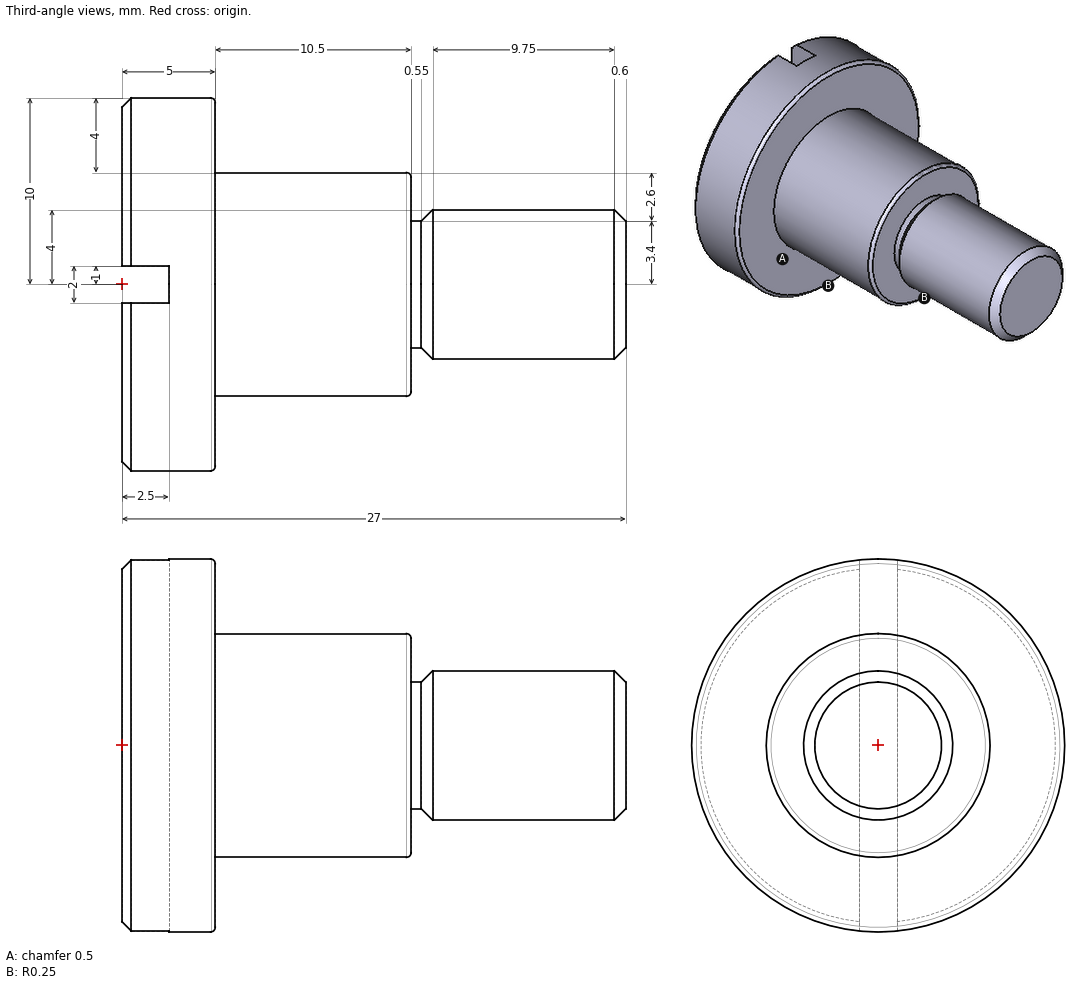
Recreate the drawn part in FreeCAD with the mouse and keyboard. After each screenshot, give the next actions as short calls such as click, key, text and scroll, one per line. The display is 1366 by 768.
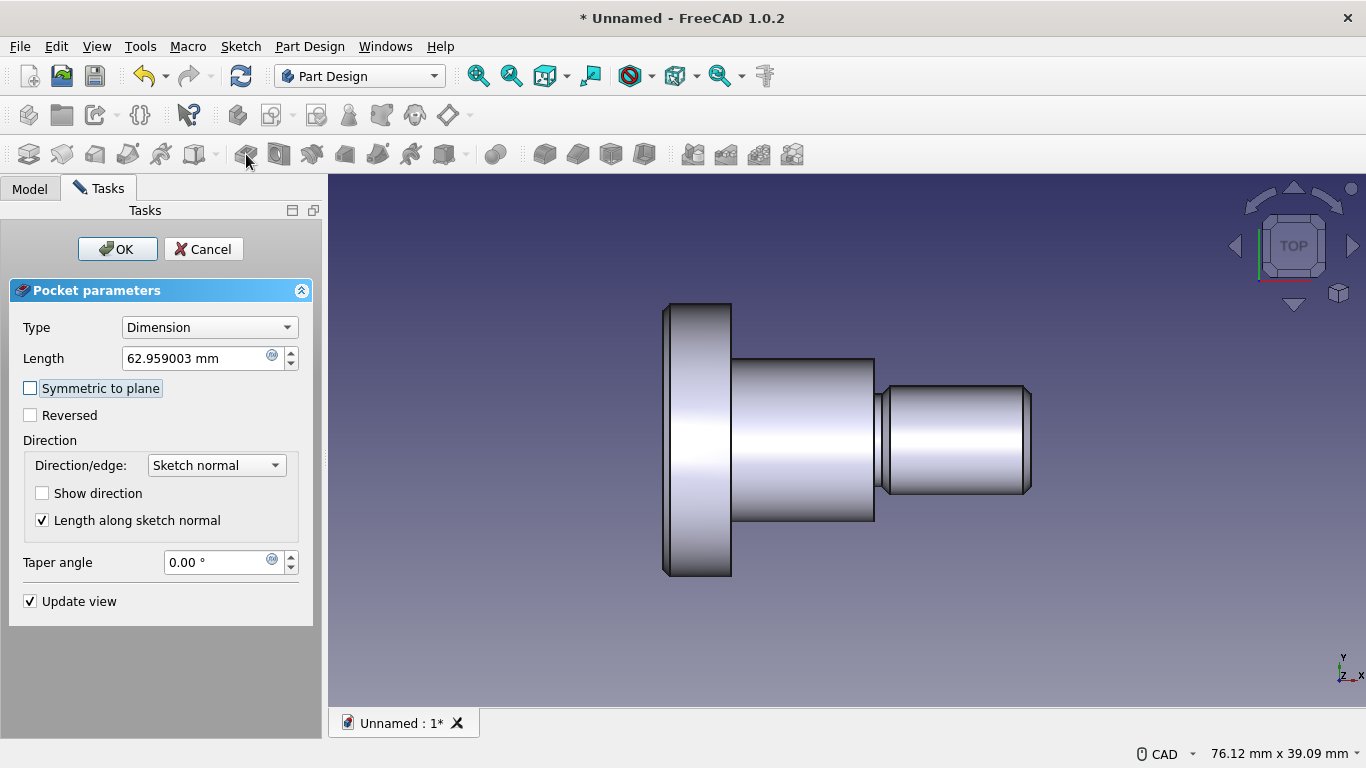
click(31, 388)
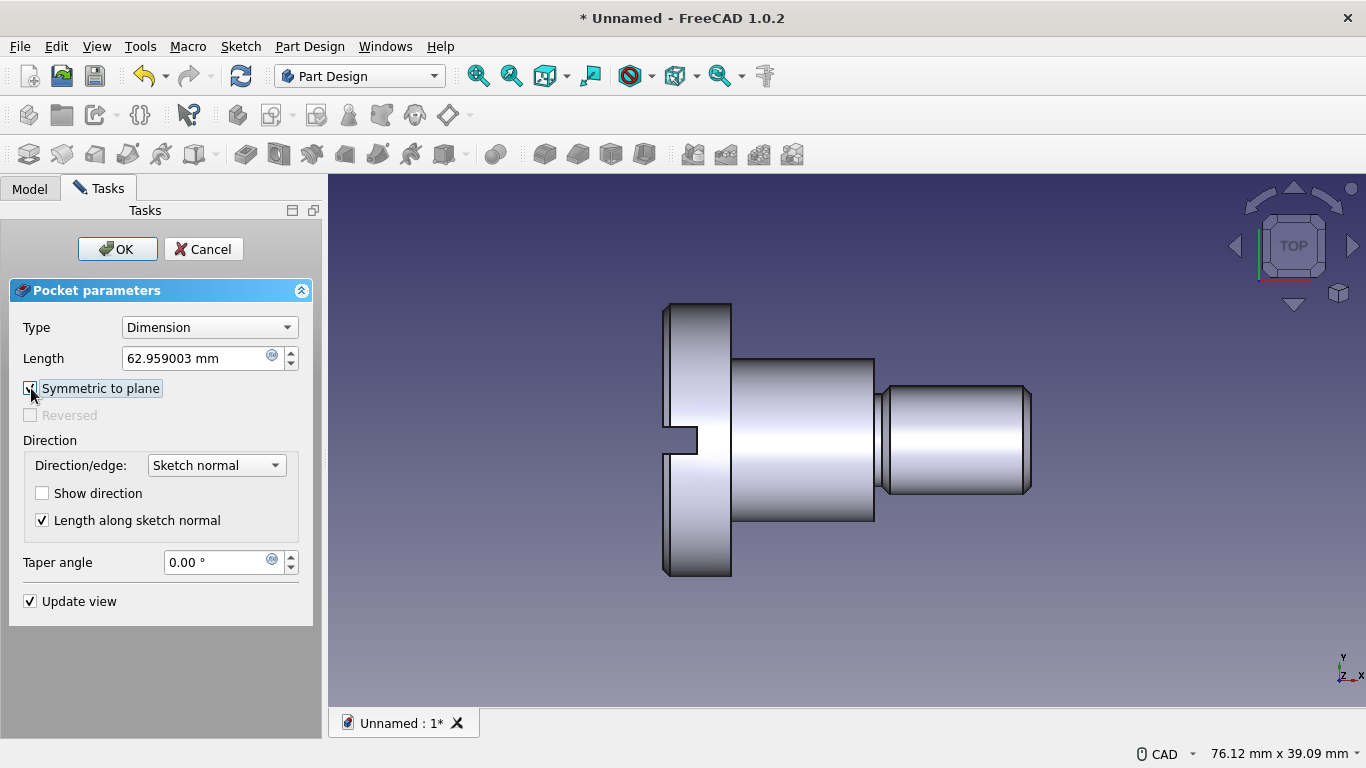
click(118, 249)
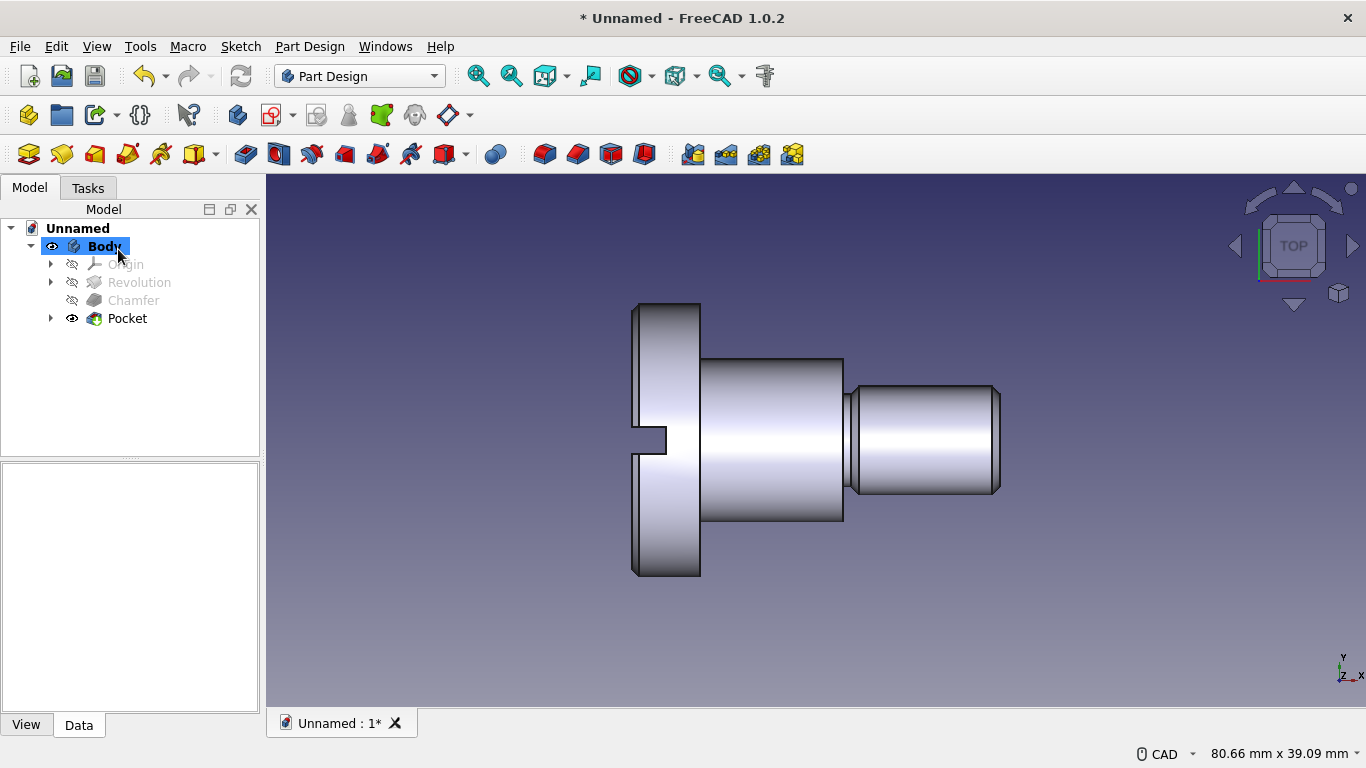
click(843, 506)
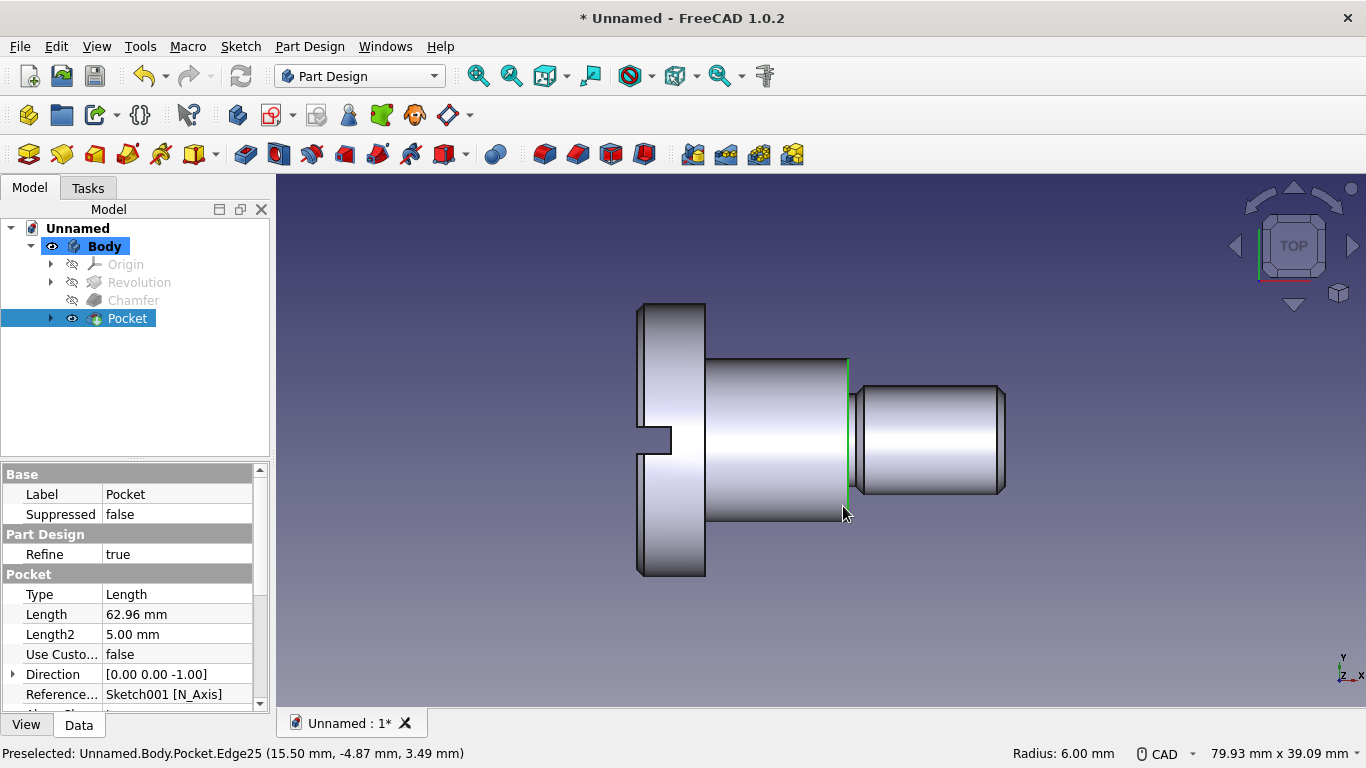
click(705, 482, ctrl)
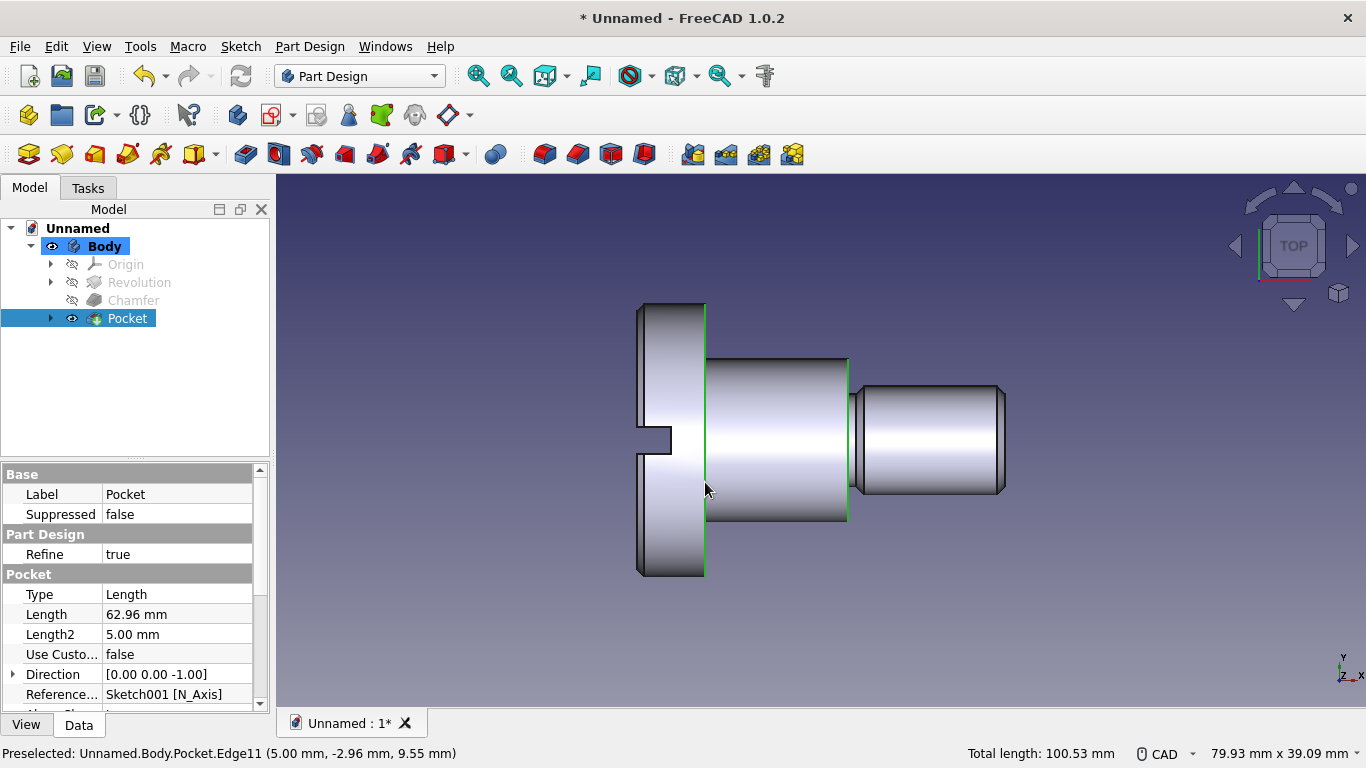
click(545, 154)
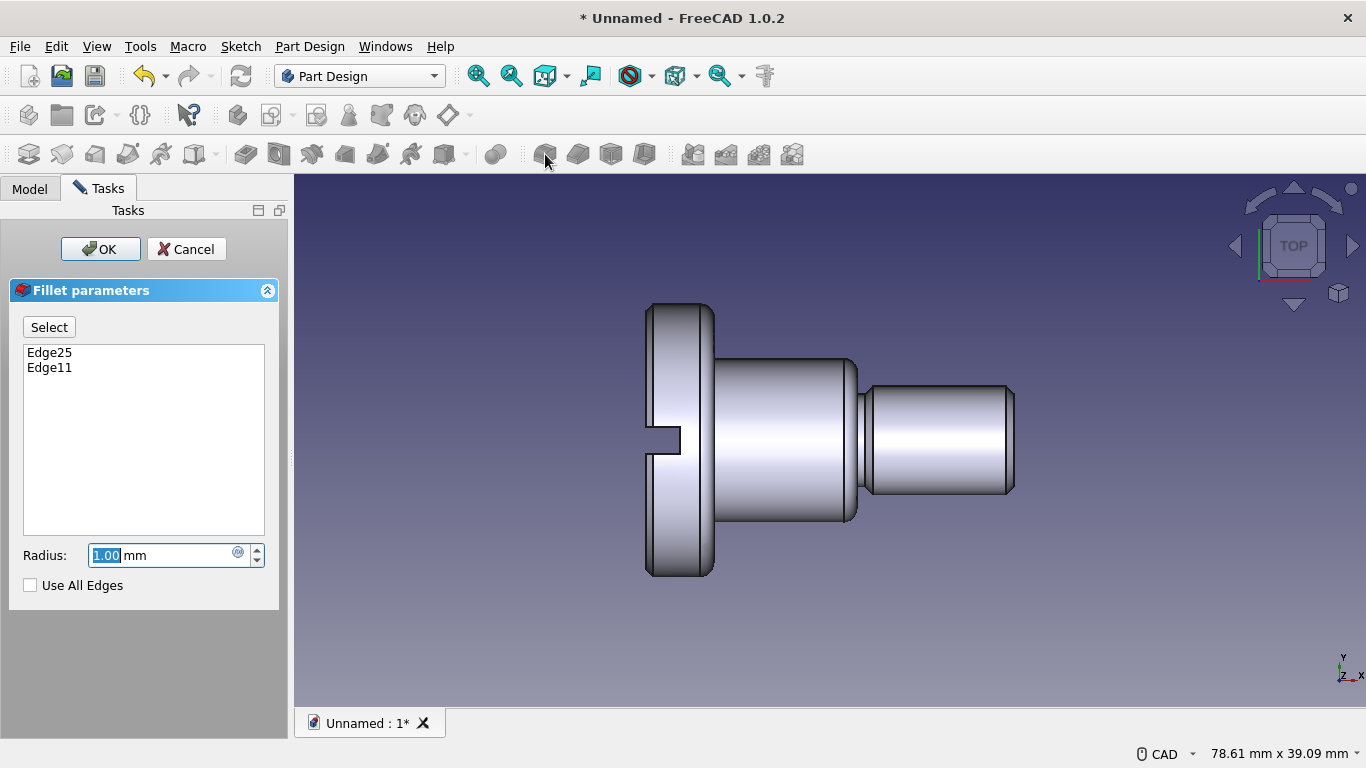
text(0.25)
key(Tab)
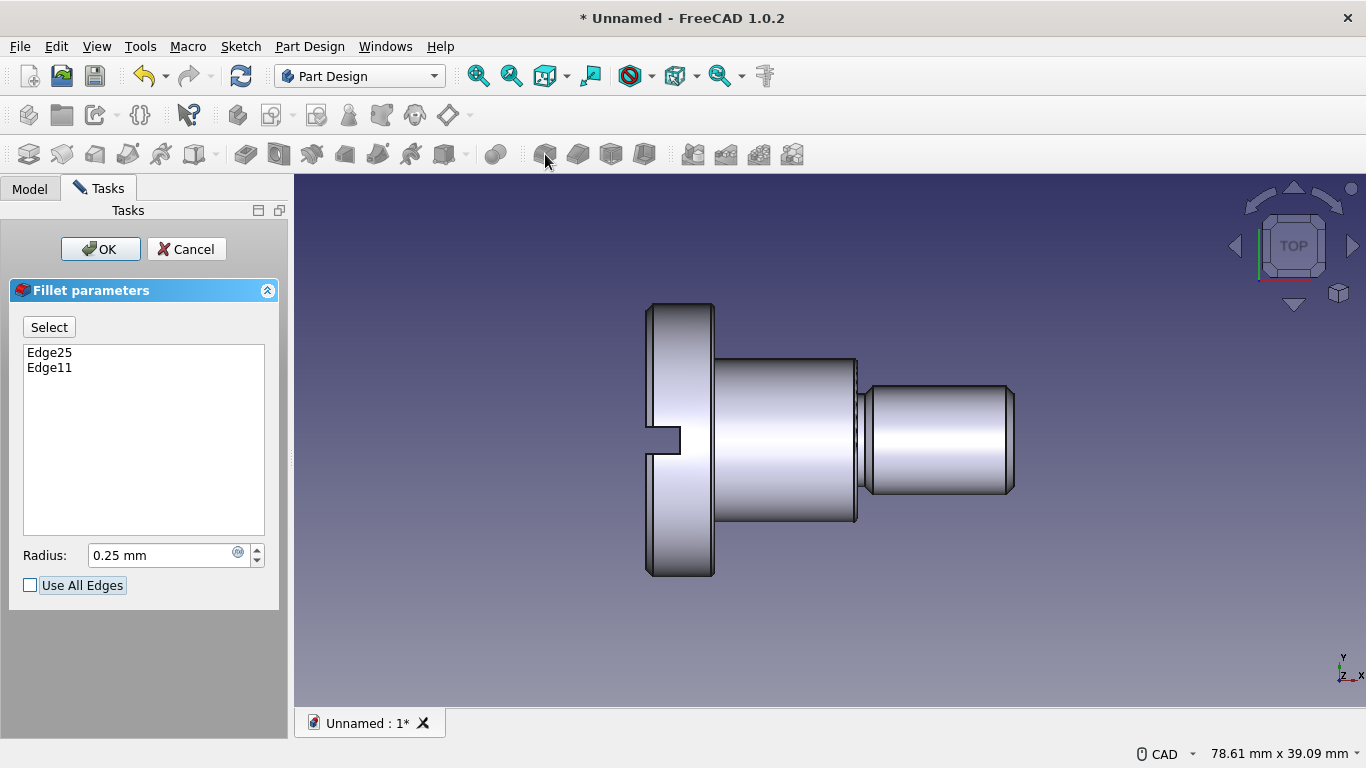
click(101, 249)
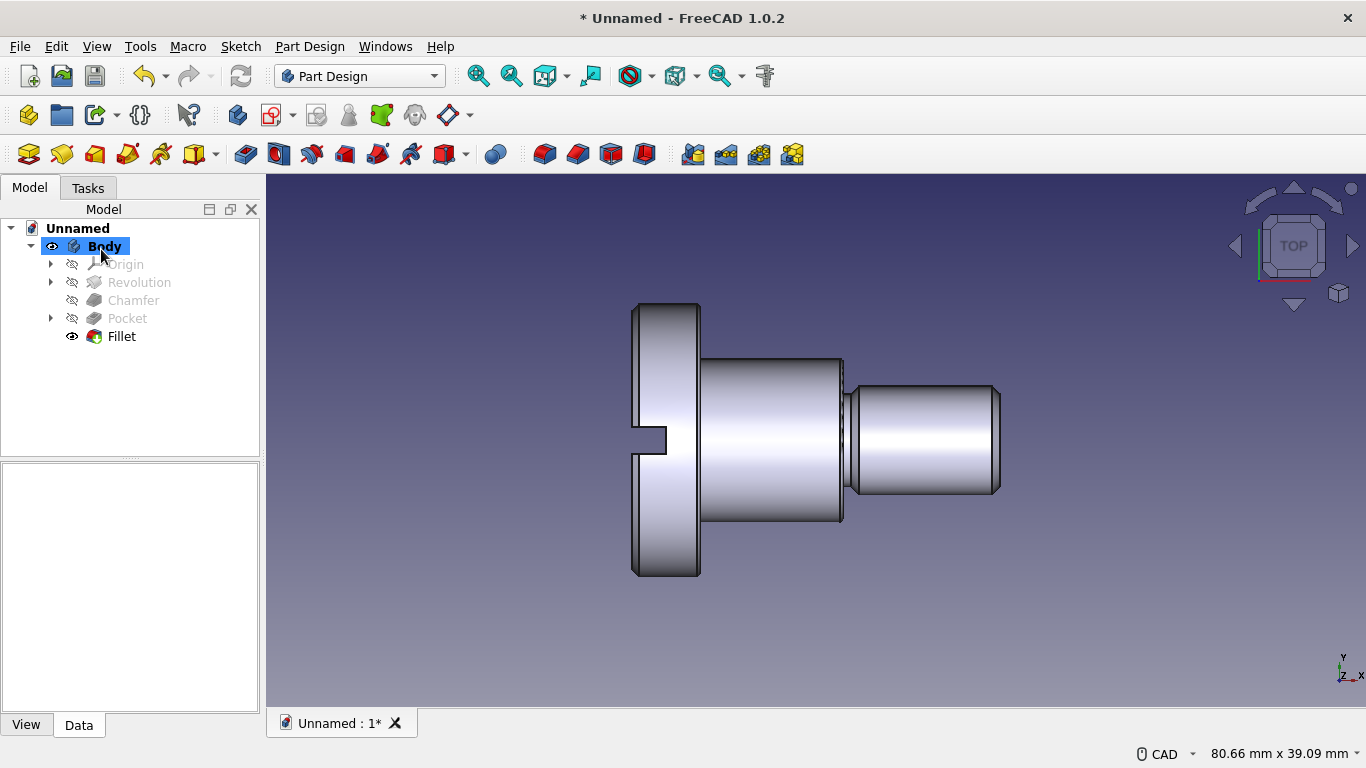
key(0)